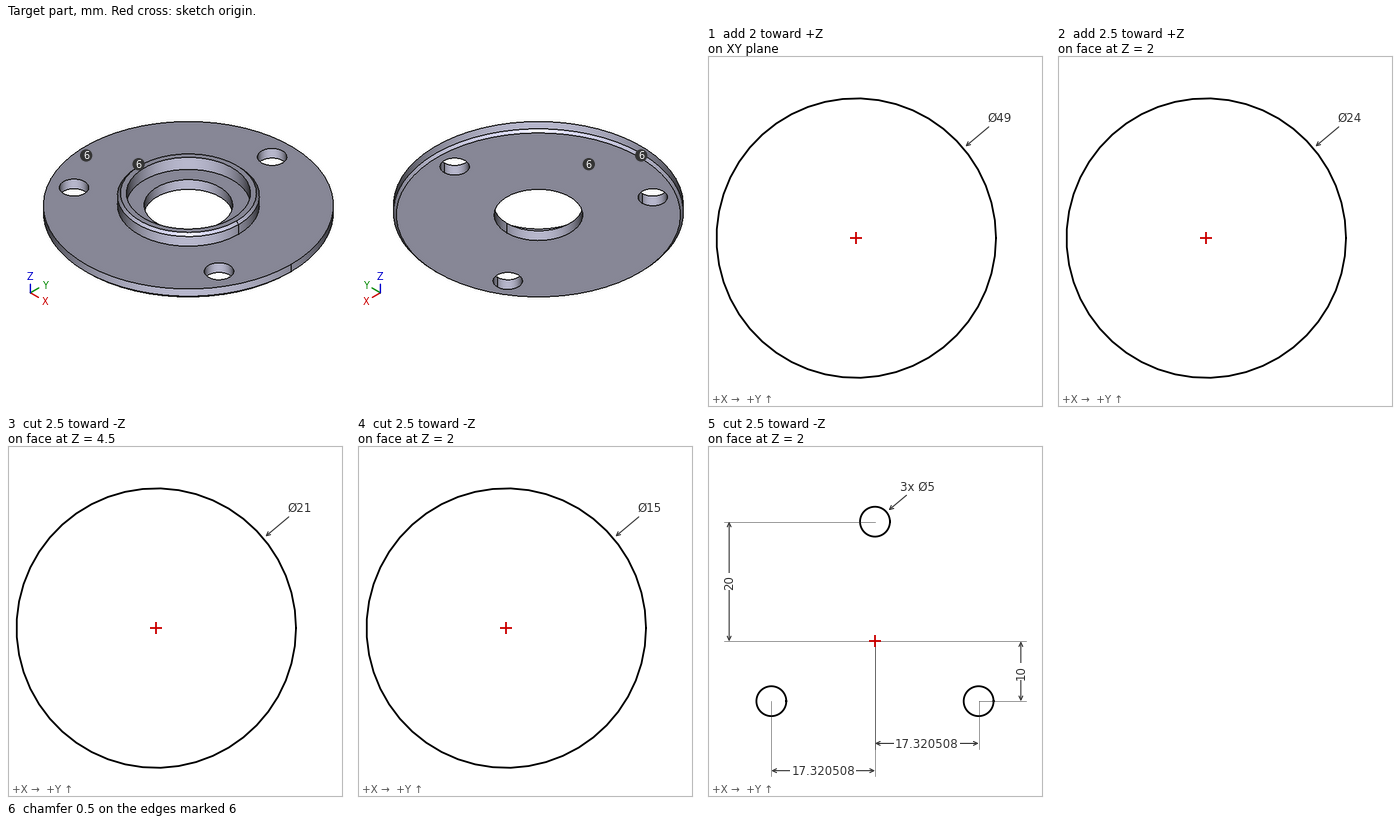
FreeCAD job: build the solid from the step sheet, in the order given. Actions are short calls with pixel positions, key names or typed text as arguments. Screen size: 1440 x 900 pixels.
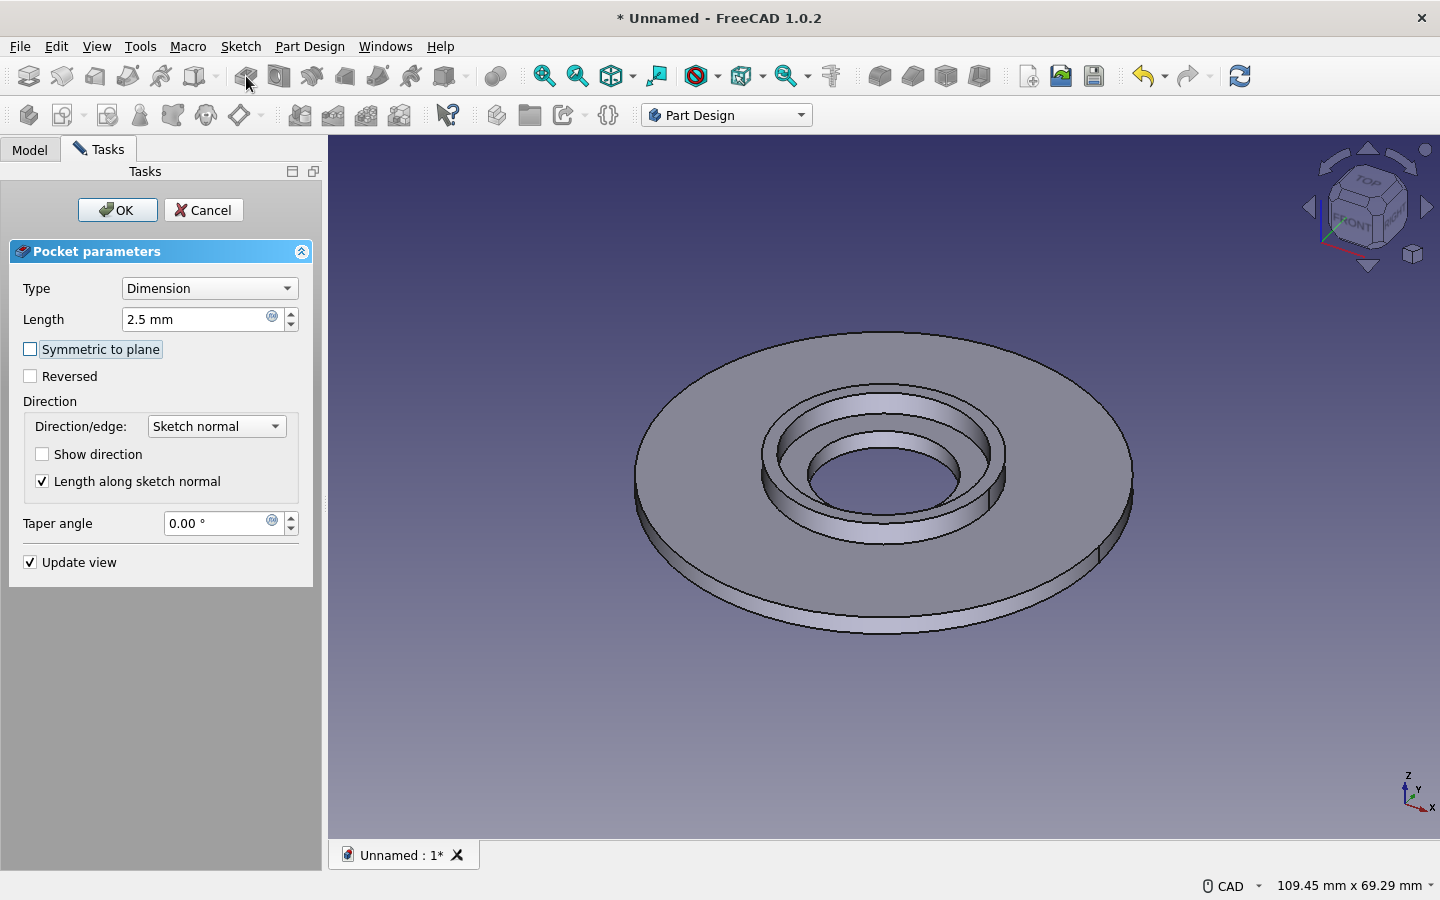
click(118, 210)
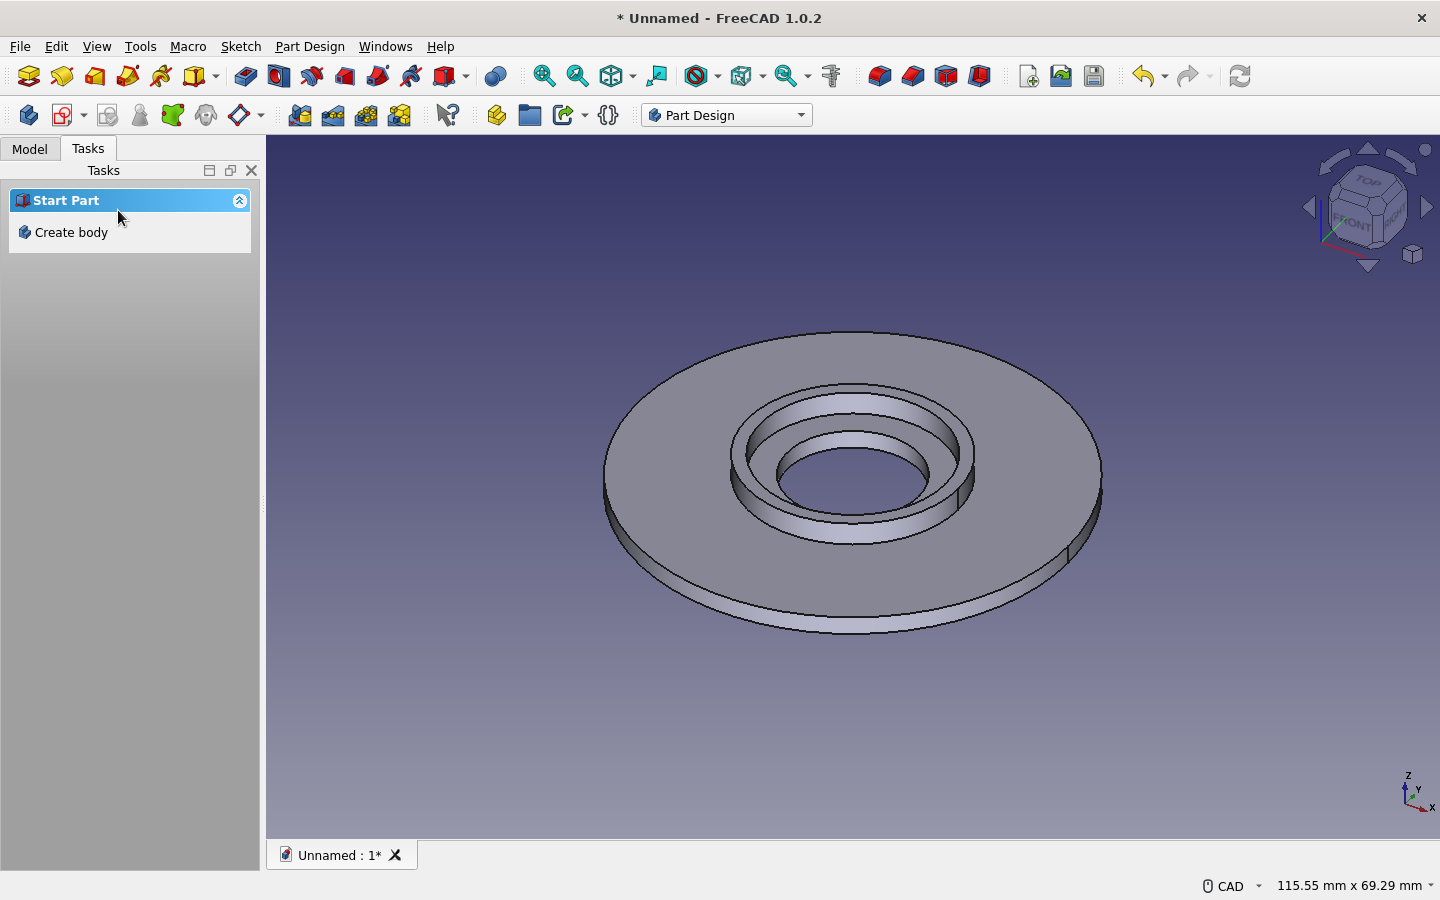
click(1047, 444)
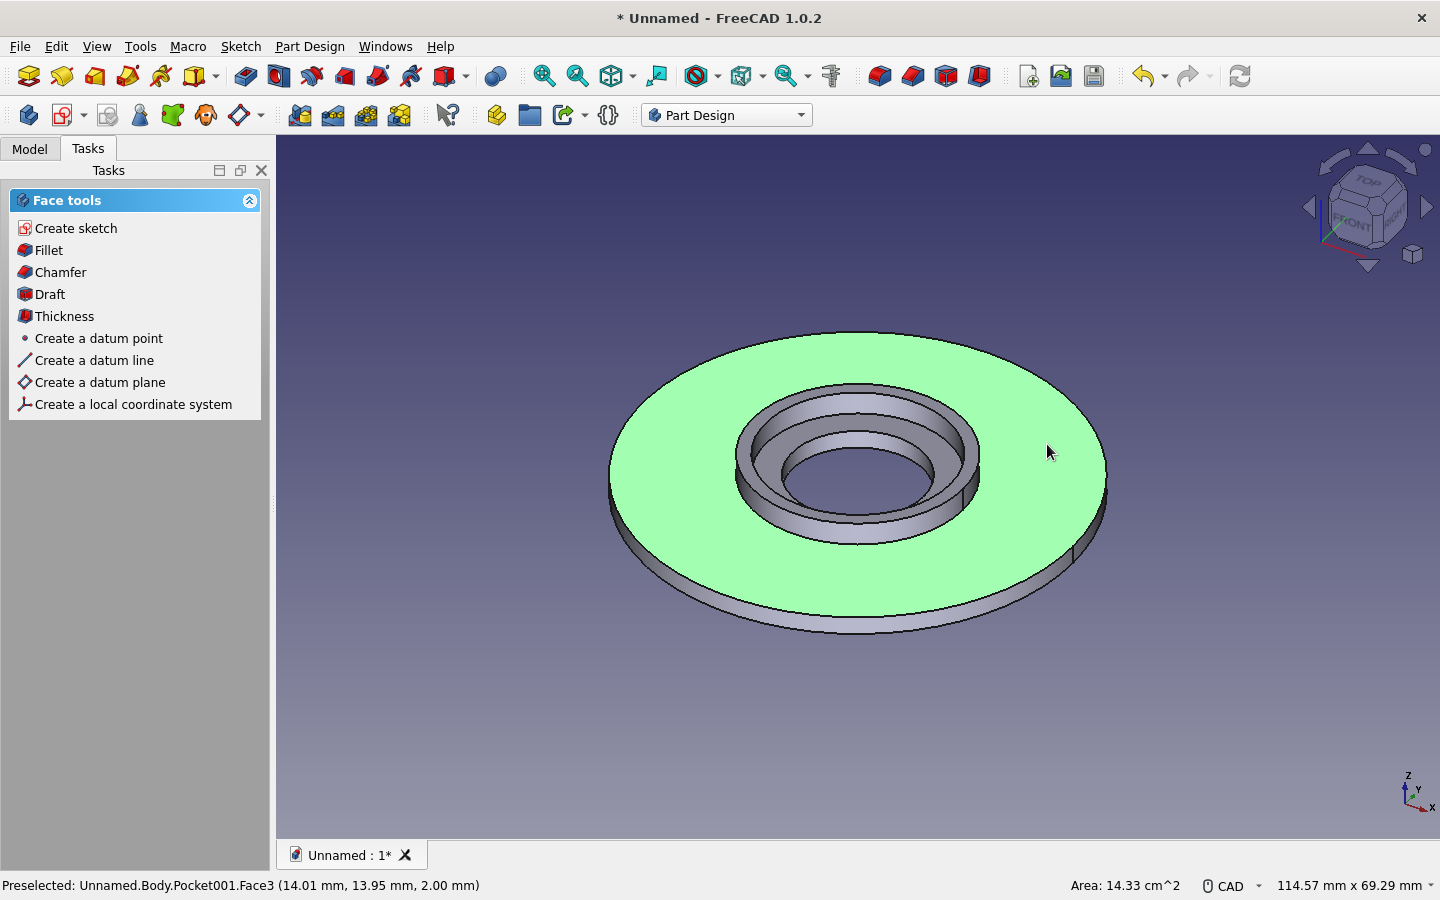
click(62, 116)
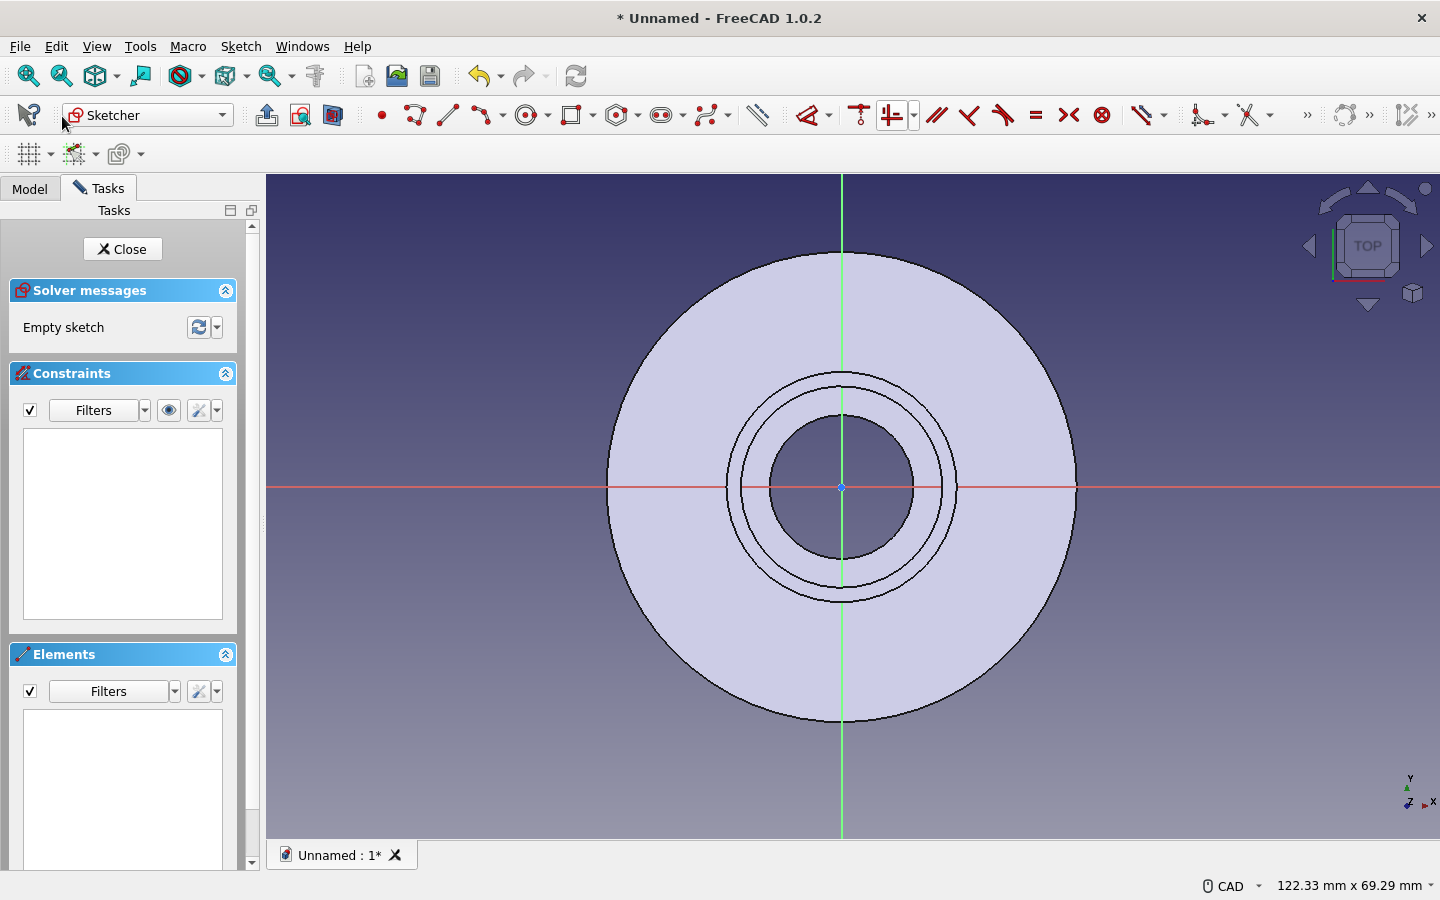
click(333, 116)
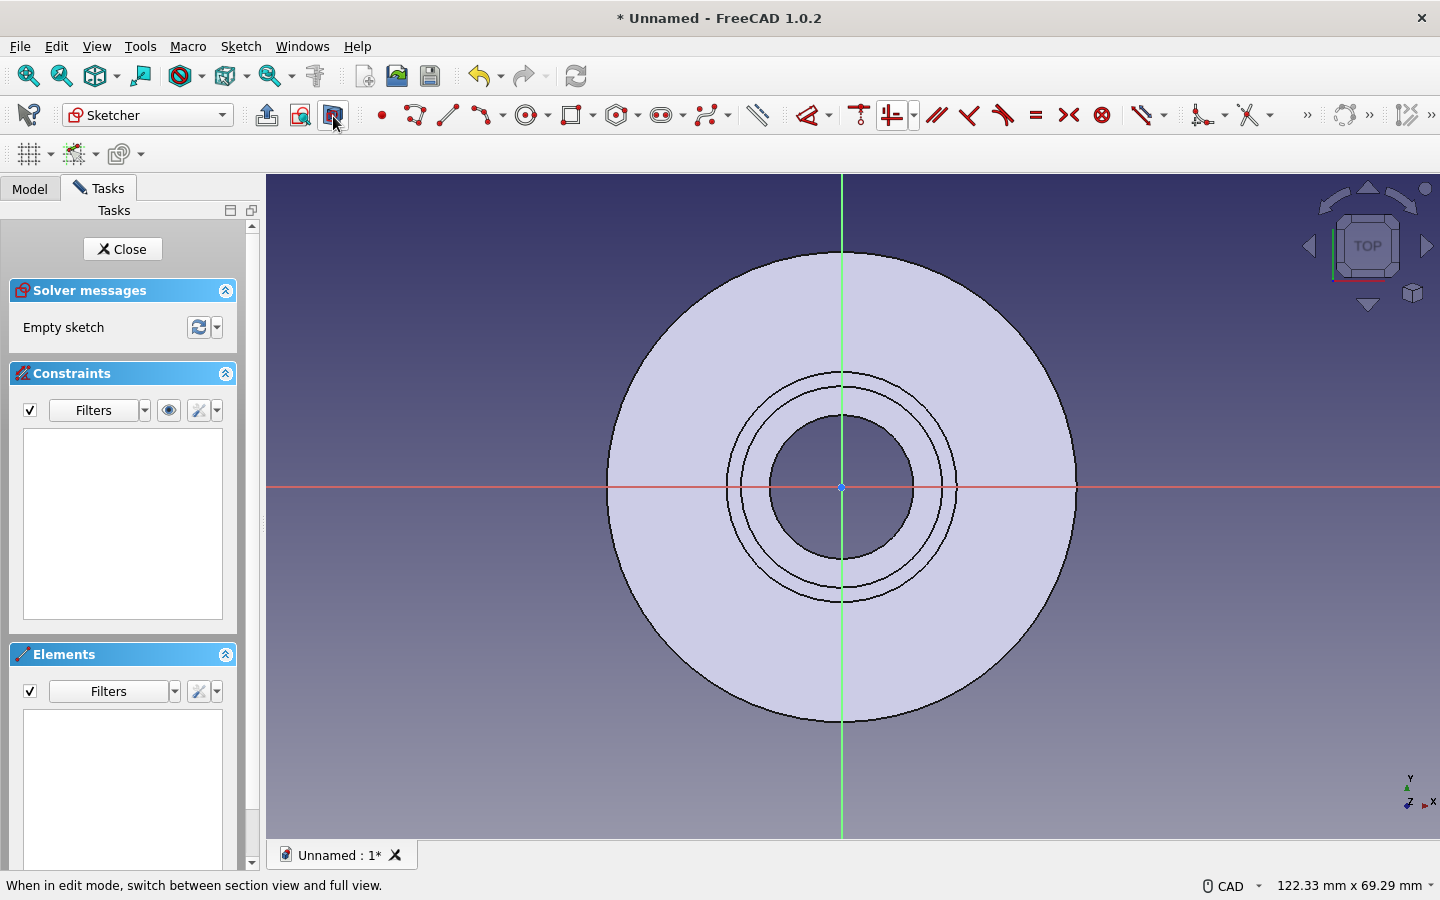
click(526, 116)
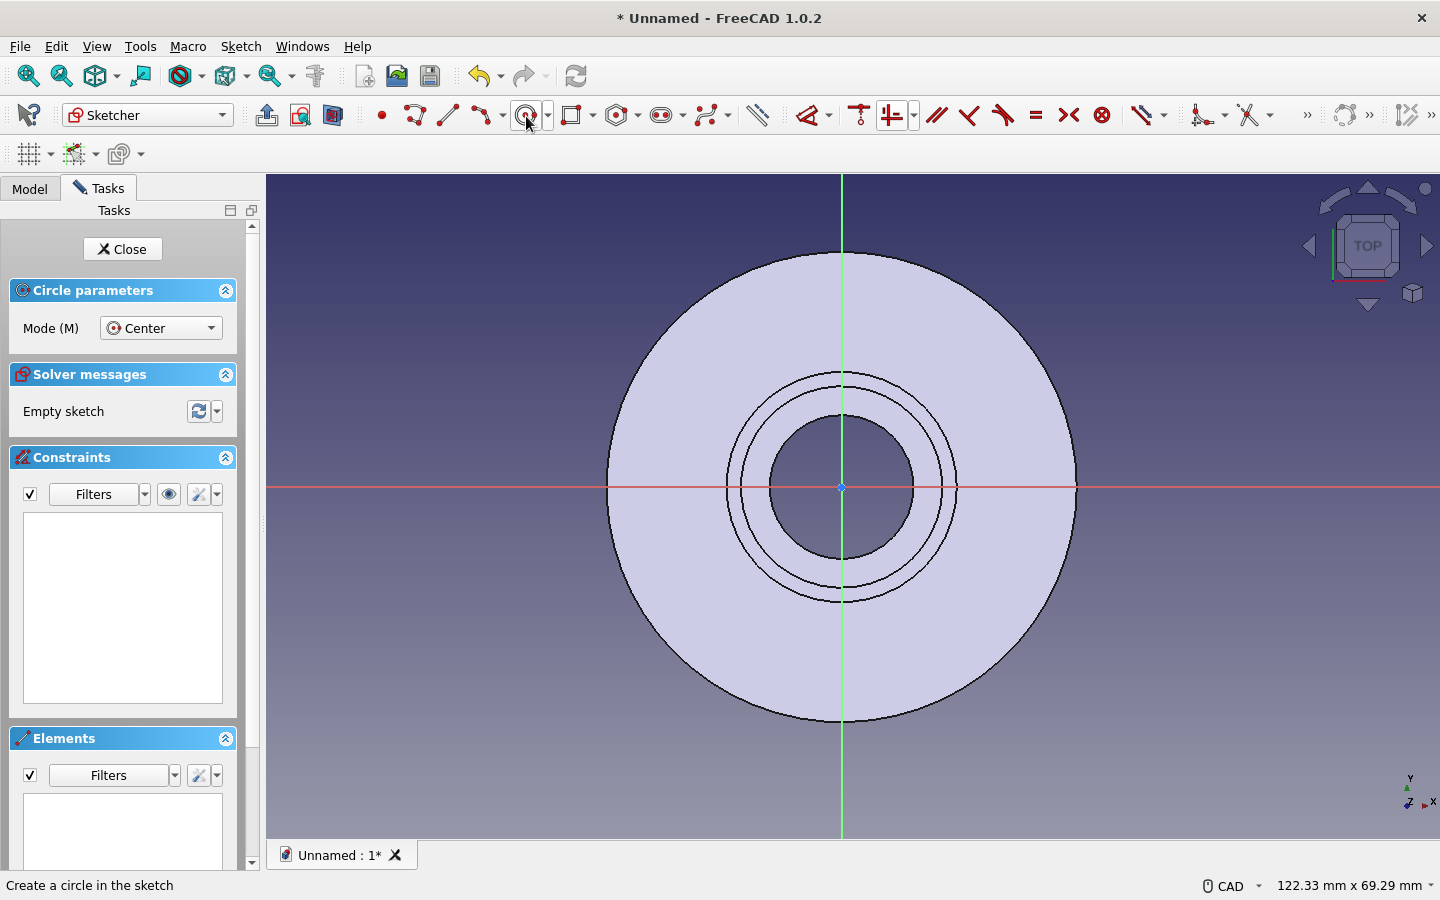
click(842, 295)
click(859, 278)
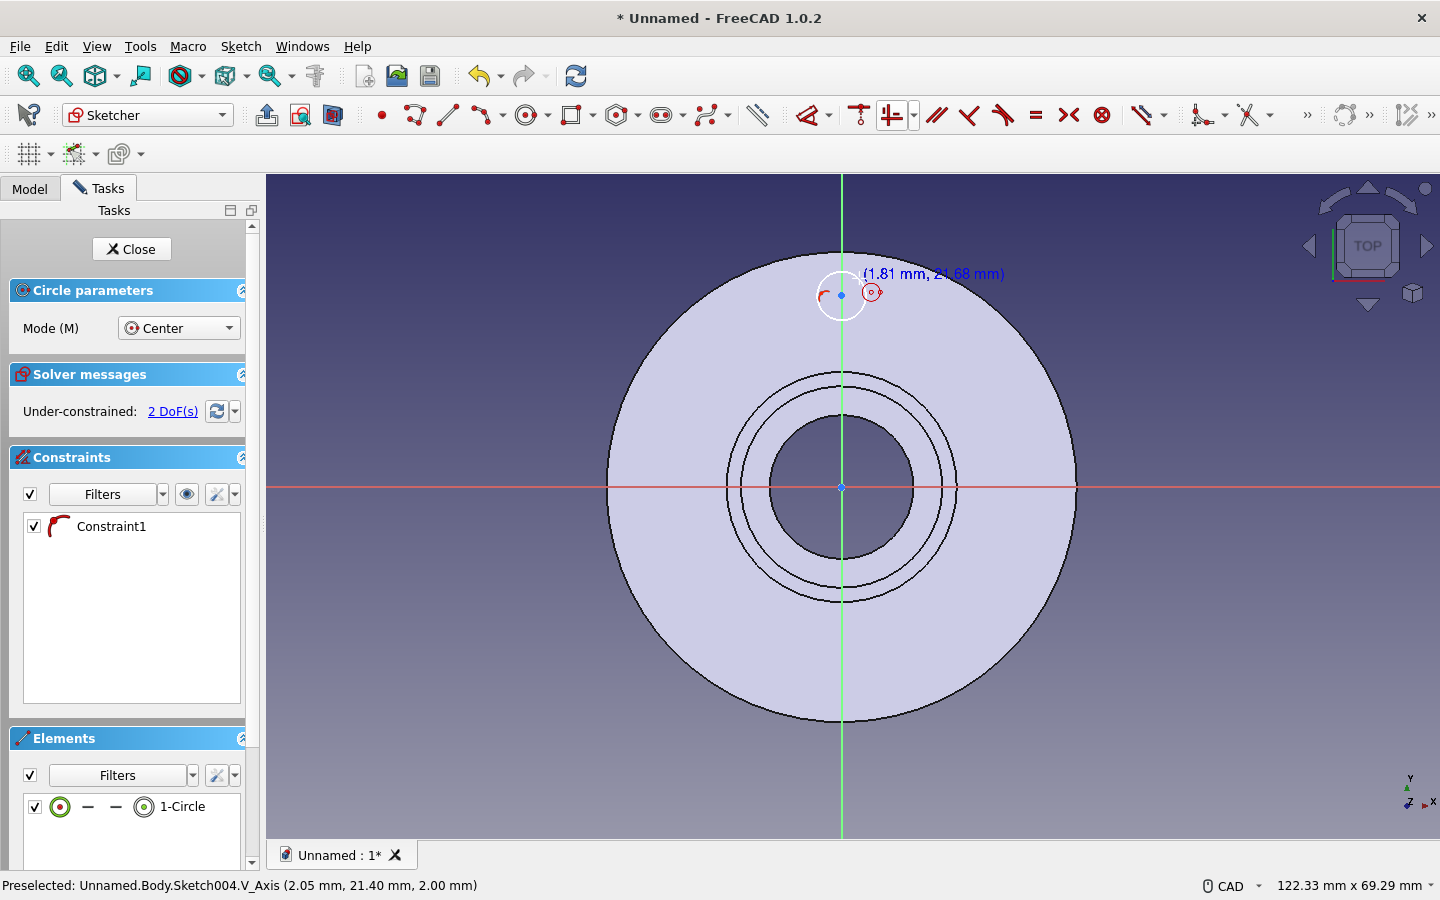
click(1008, 583)
click(1025, 566)